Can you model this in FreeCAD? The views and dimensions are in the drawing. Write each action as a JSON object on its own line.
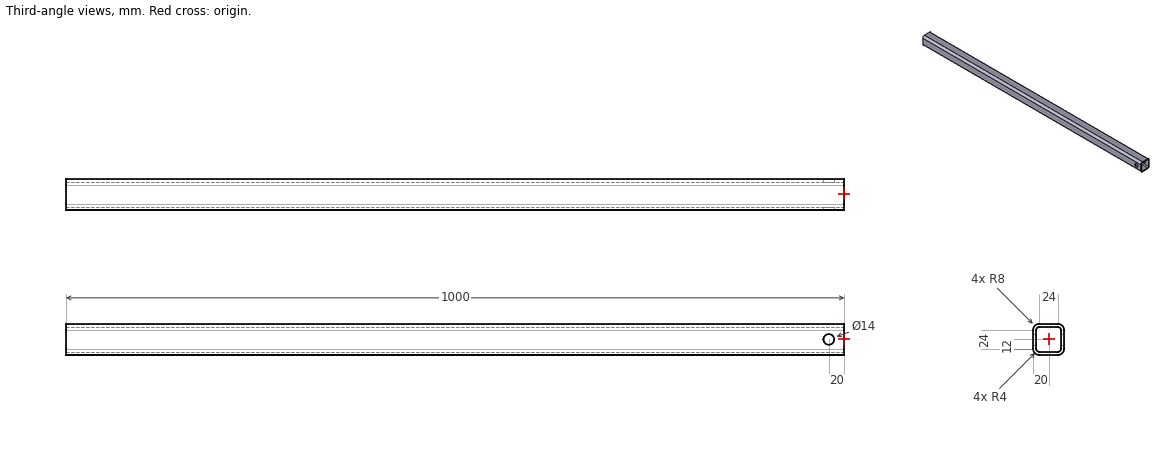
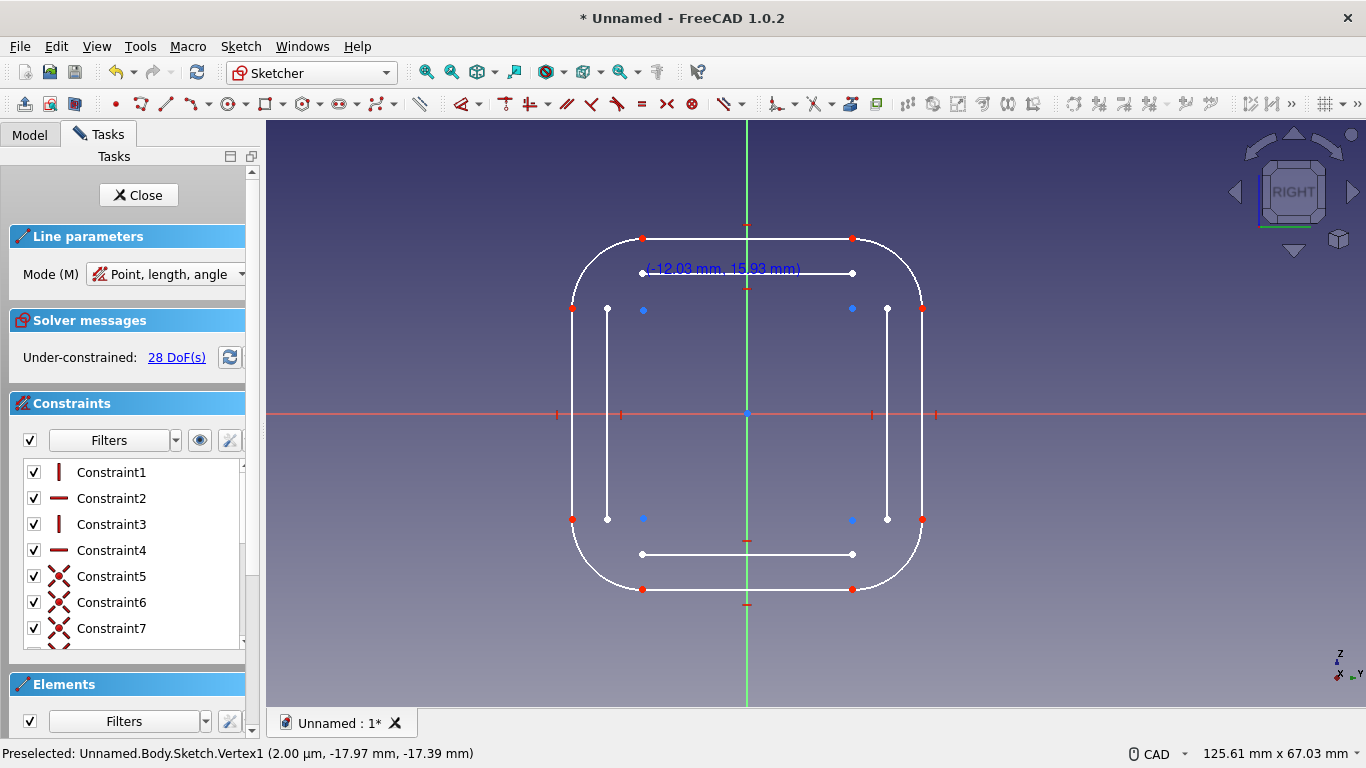
{"action": "left_click", "coordinate": [190, 104]}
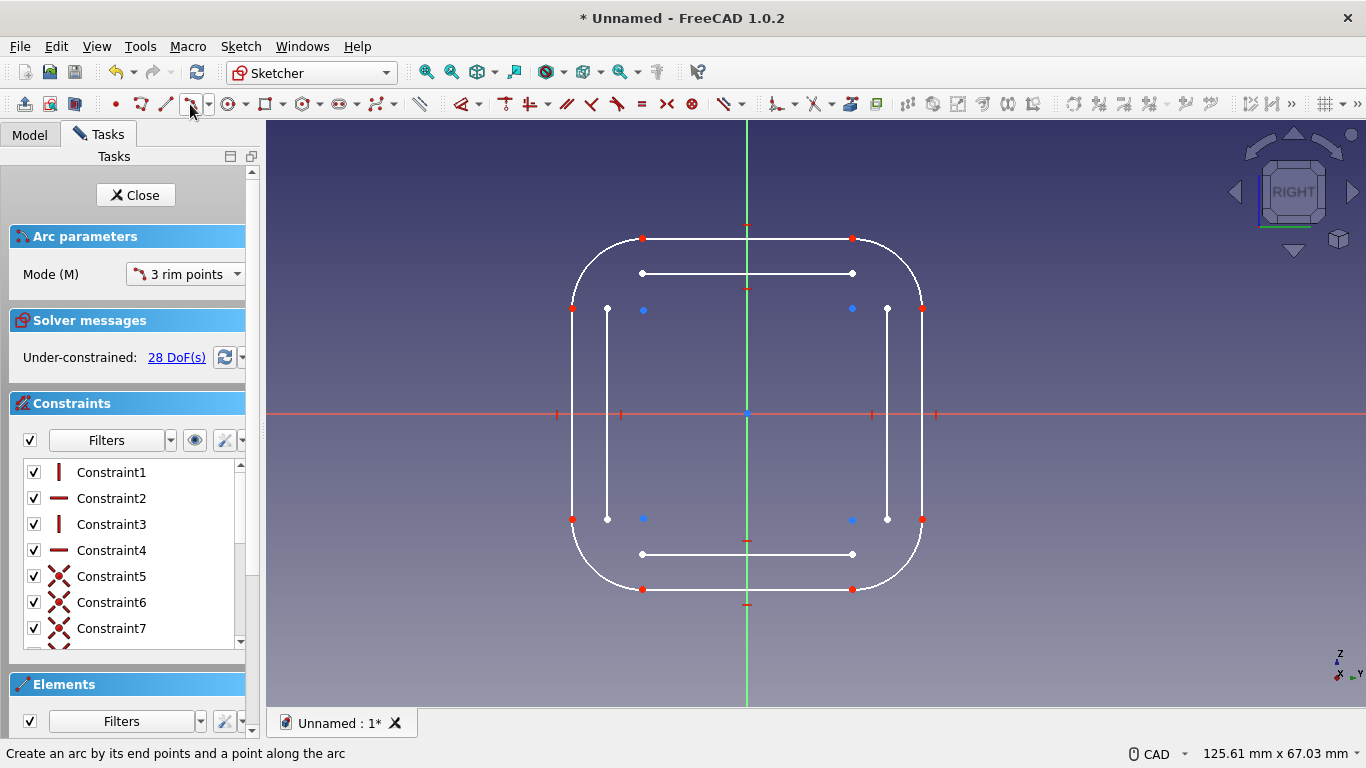
{"action": "left_click", "coordinate": [607, 520]}
{"action": "left_click", "coordinate": [642, 555]}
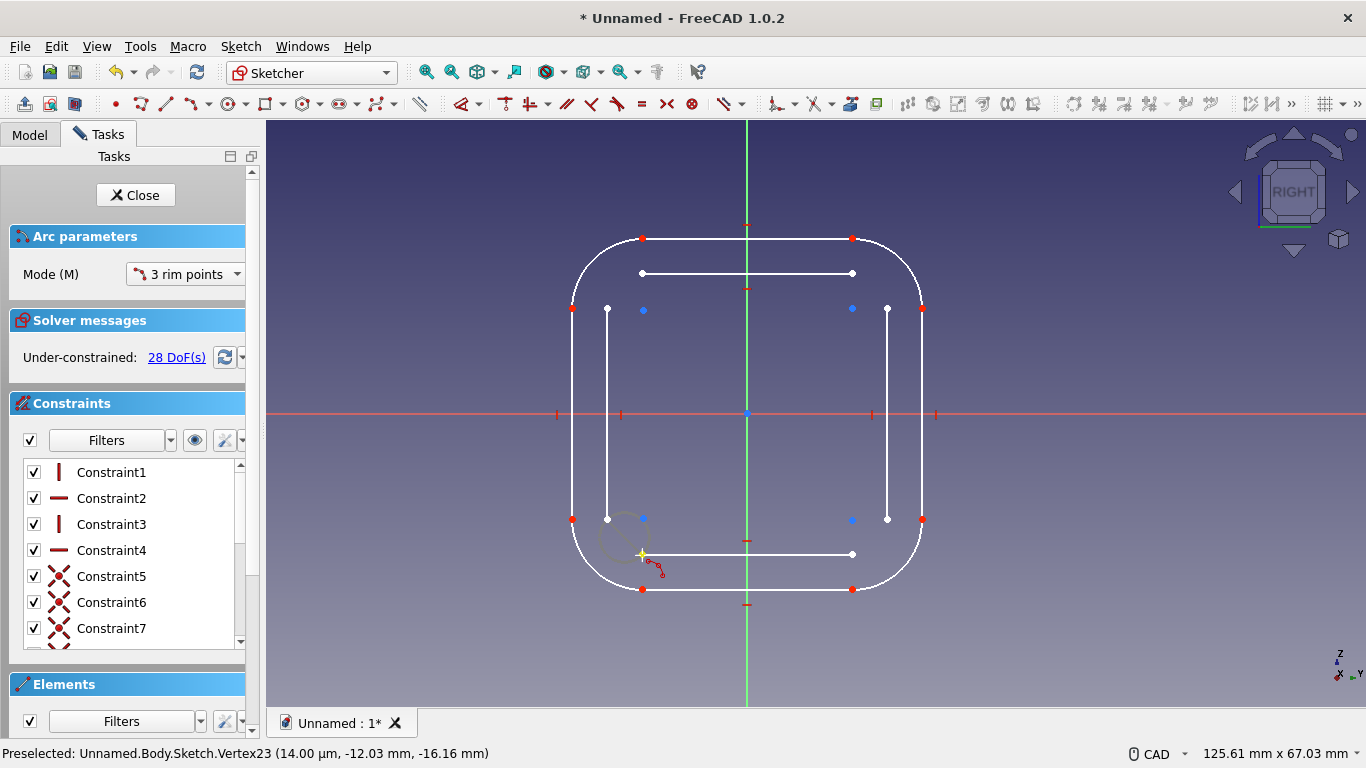
{"action": "scroll", "coordinate": [617, 543], "scroll_direction": "up", "scroll_amount": 3}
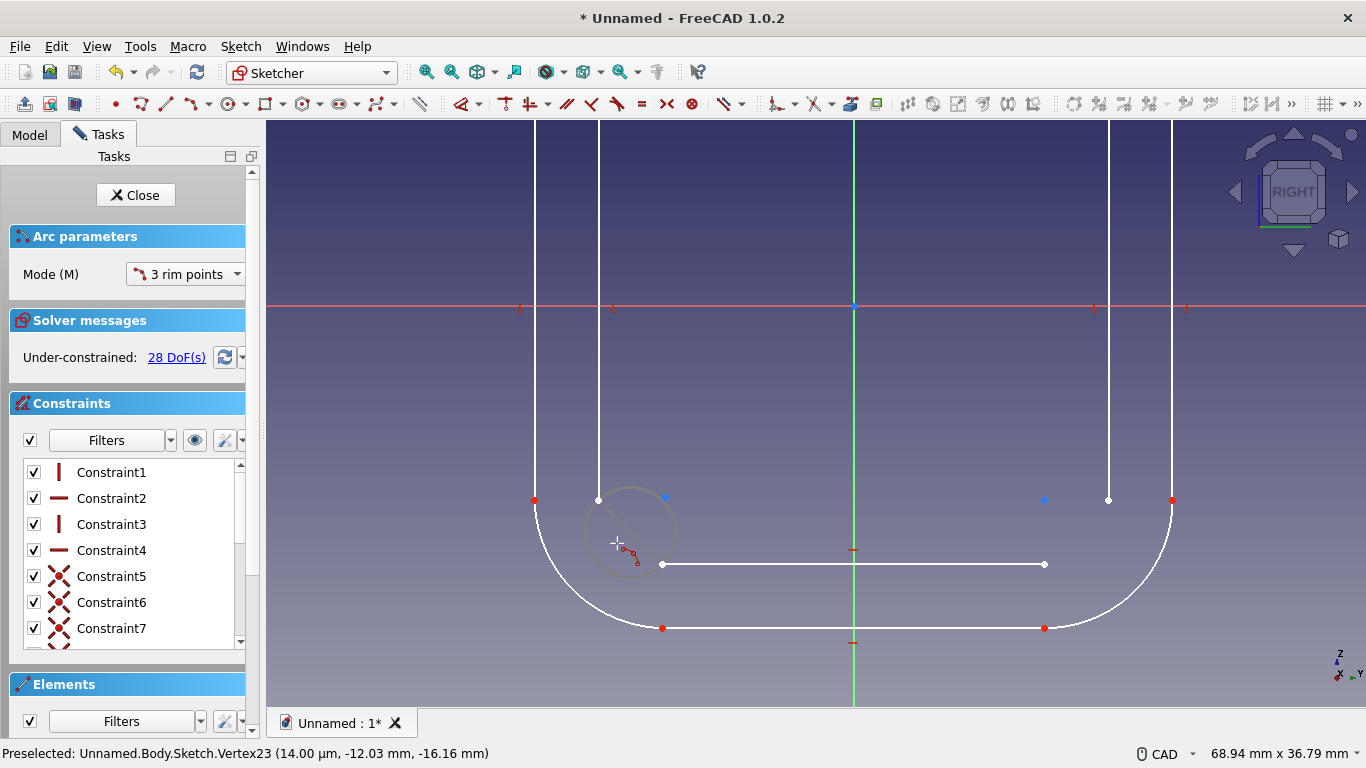
{"action": "left_click", "coordinate": [618, 543]}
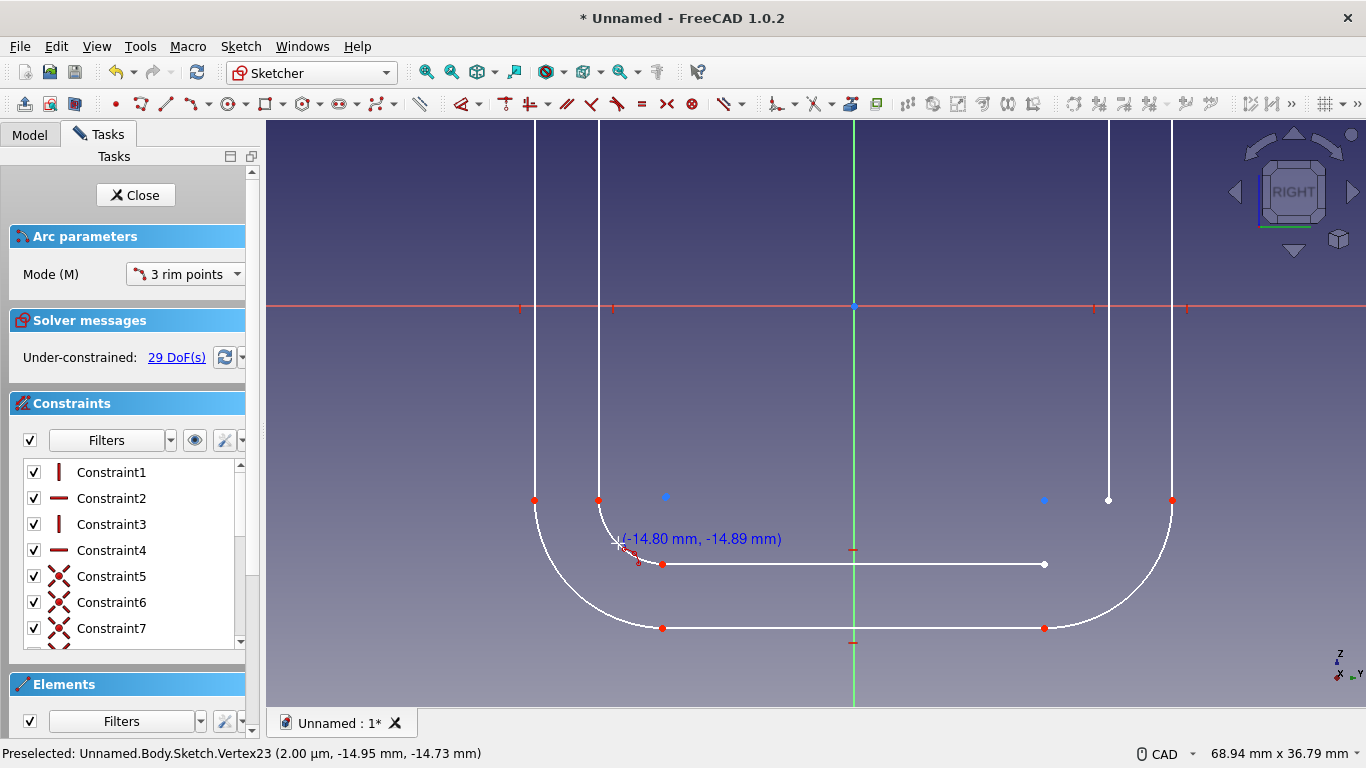
{"action": "left_click", "coordinate": [1045, 564]}
{"action": "left_click", "coordinate": [1109, 500]}
{"action": "left_click", "coordinate": [1091, 543]}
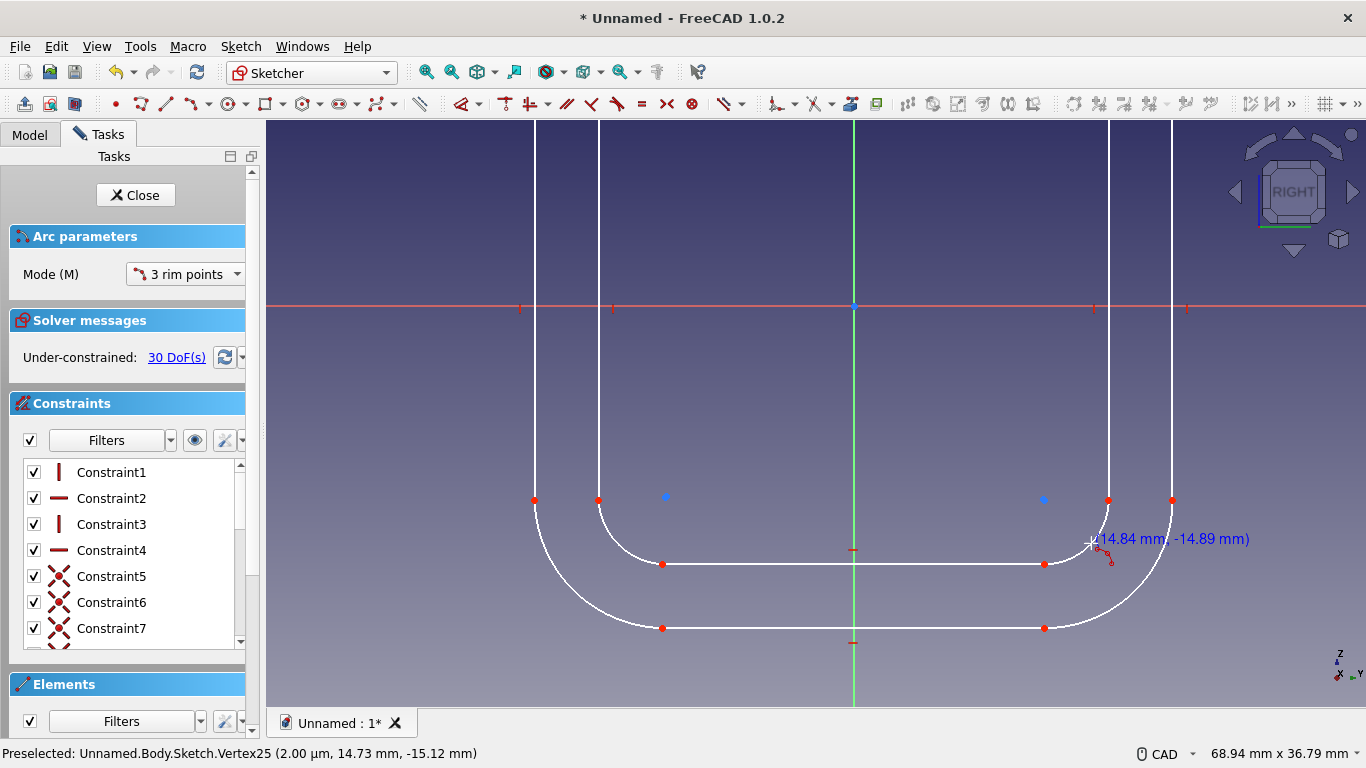
{"action": "scroll", "coordinate": [618, 544], "scroll_direction": "down", "scroll_amount": 3}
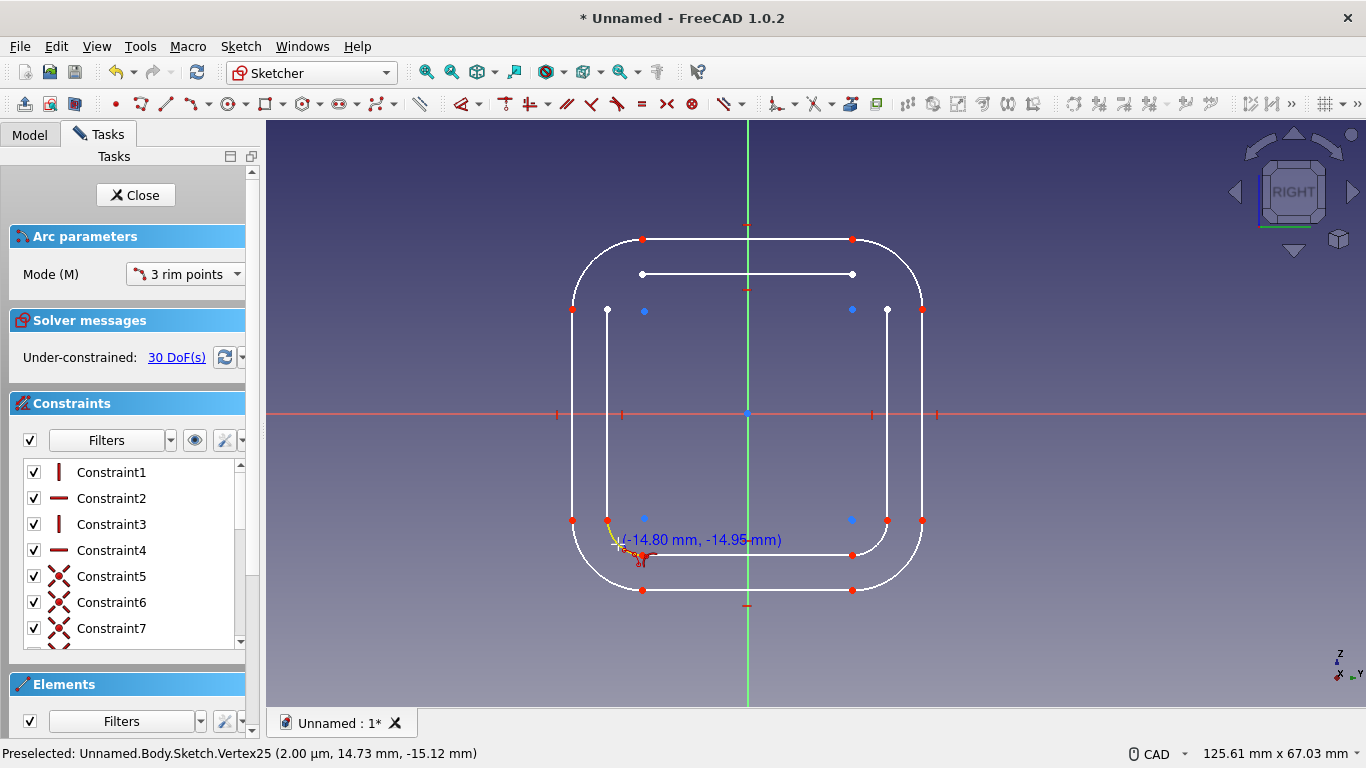
{"action": "left_click", "coordinate": [887, 309]}
{"action": "left_click", "coordinate": [852, 274]}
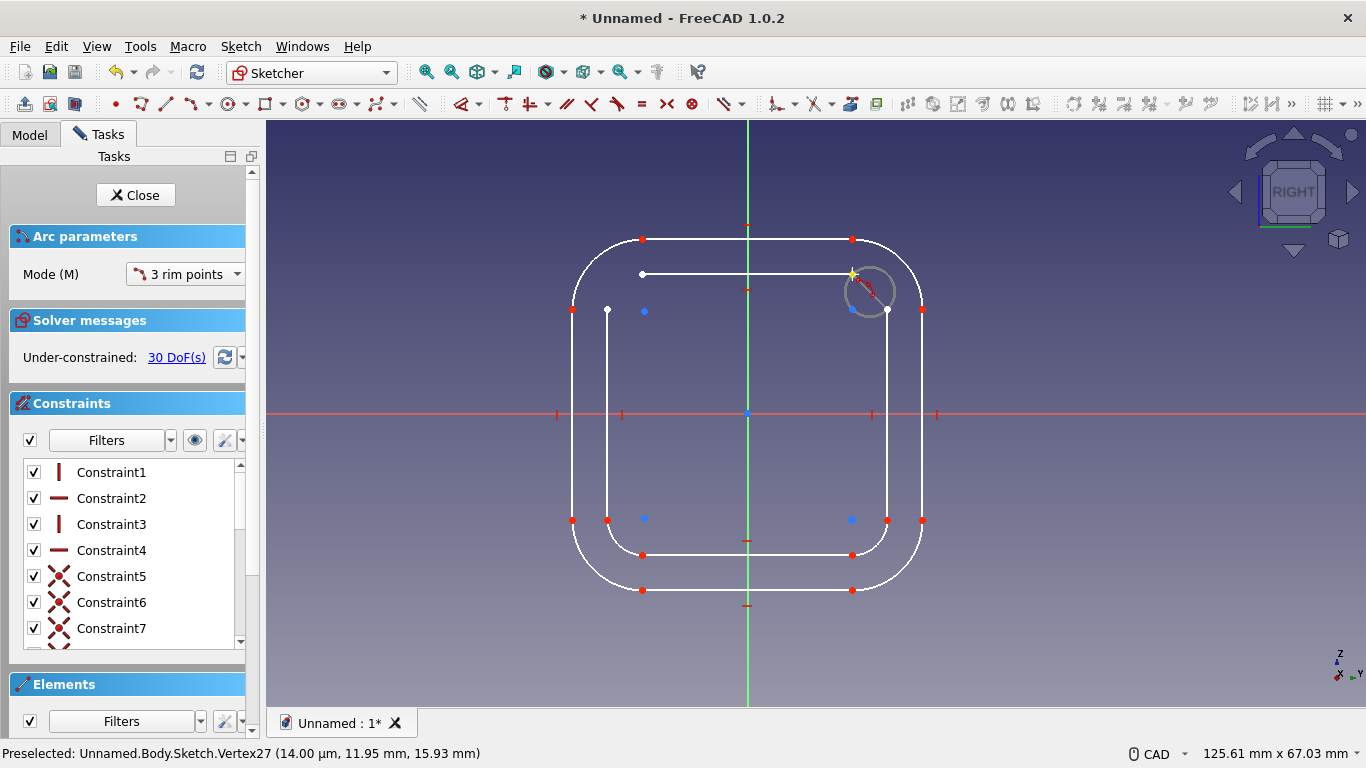
{"action": "scroll", "coordinate": [878, 284], "scroll_direction": "up", "scroll_amount": 3}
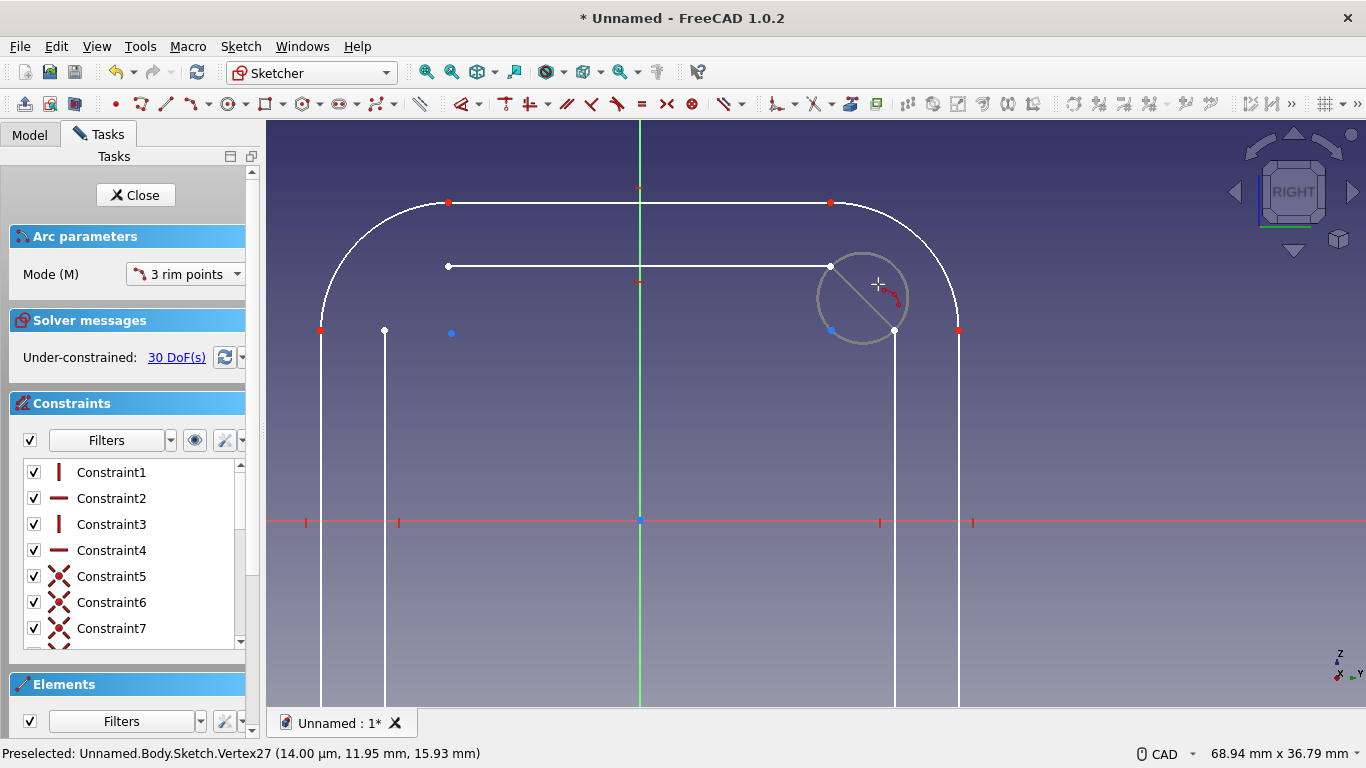
{"action": "left_click", "coordinate": [877, 284]}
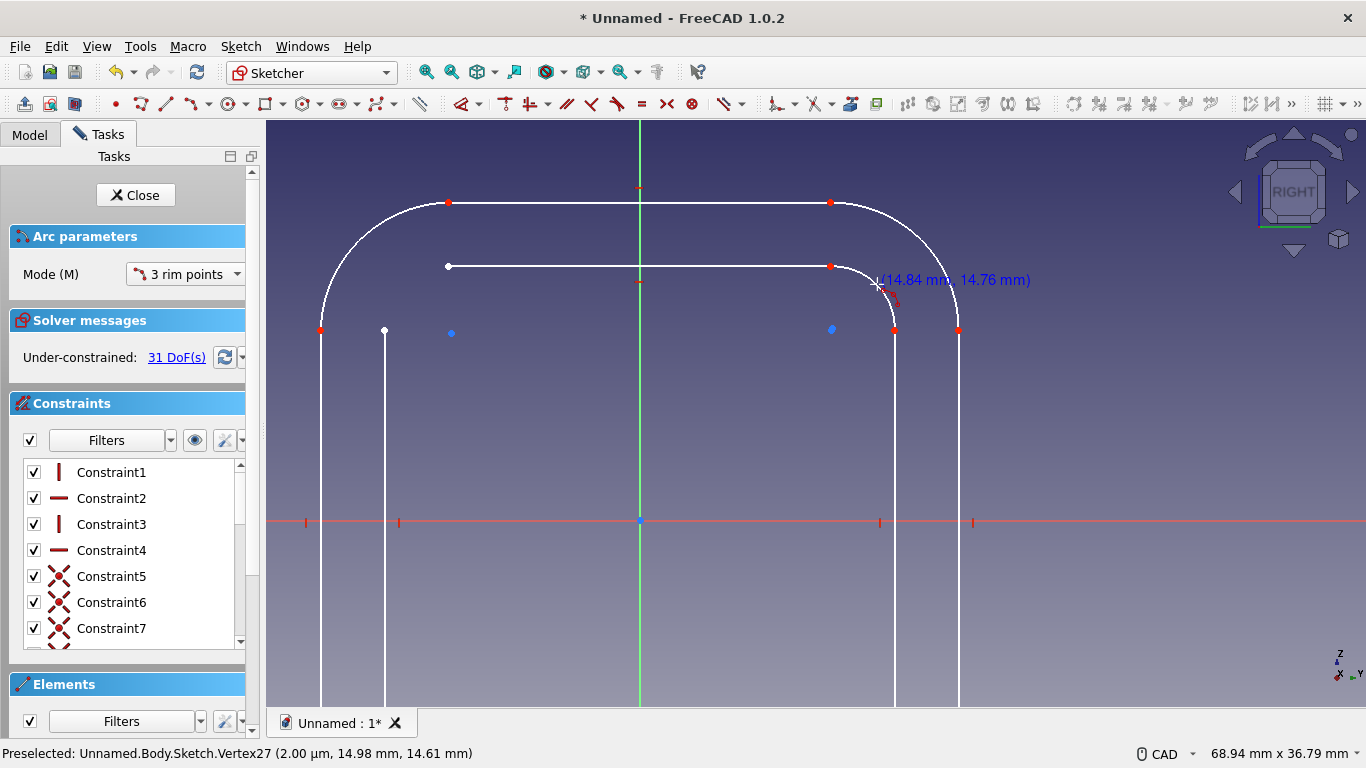
{"action": "left_click", "coordinate": [448, 266]}
{"action": "left_click", "coordinate": [385, 330]}
{"action": "left_click", "coordinate": [404, 284]}
{"action": "key", "text": "Escape"}